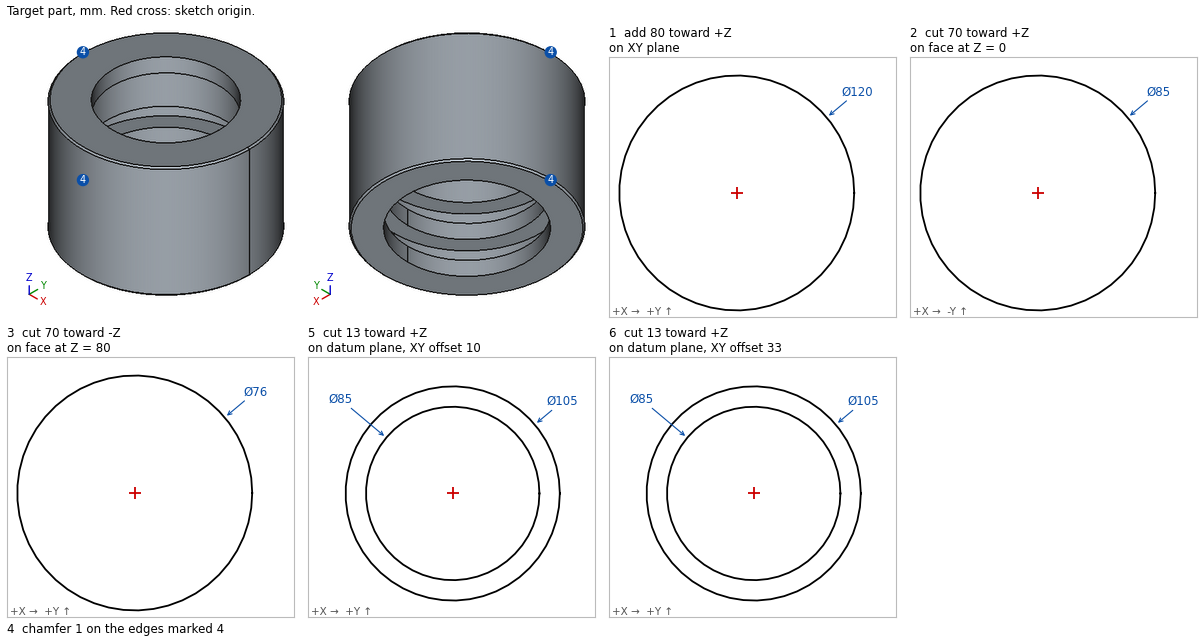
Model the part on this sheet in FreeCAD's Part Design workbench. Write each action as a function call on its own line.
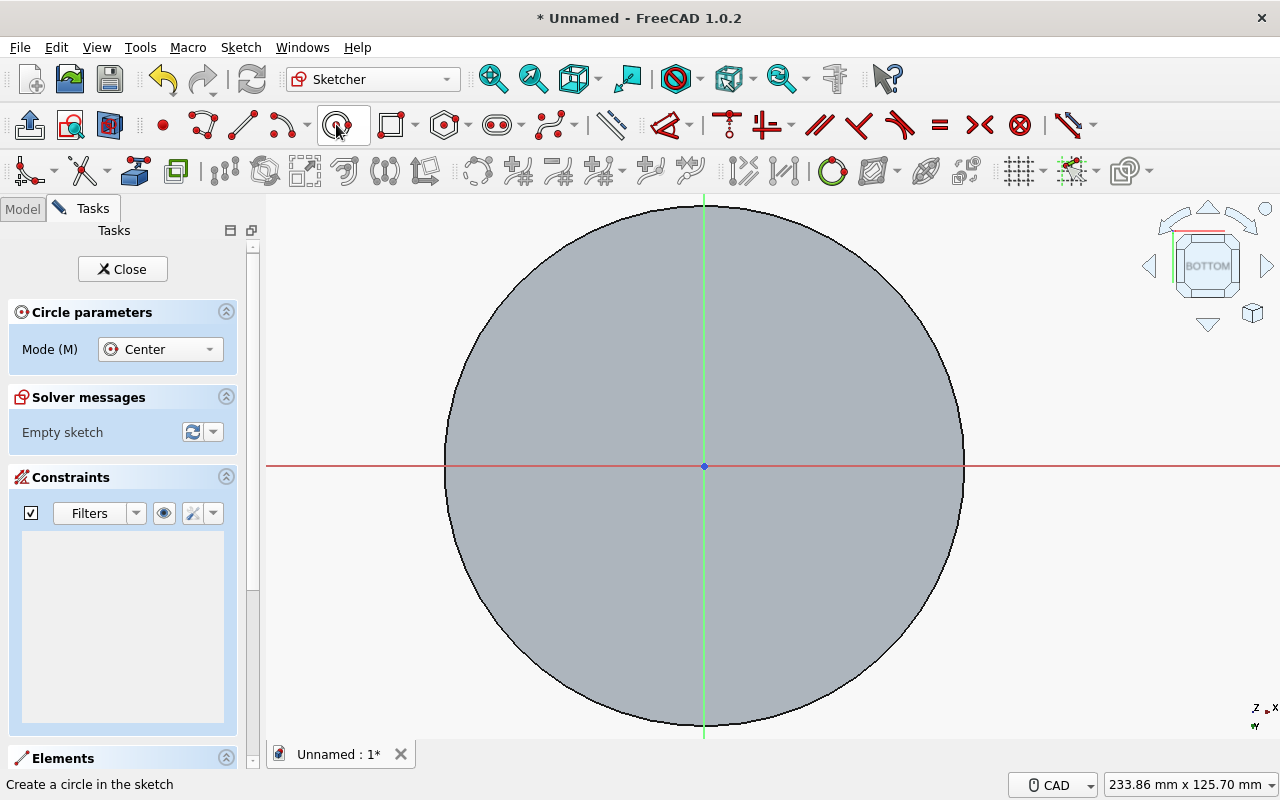
click(704, 466)
click(835, 336)
key(Escape)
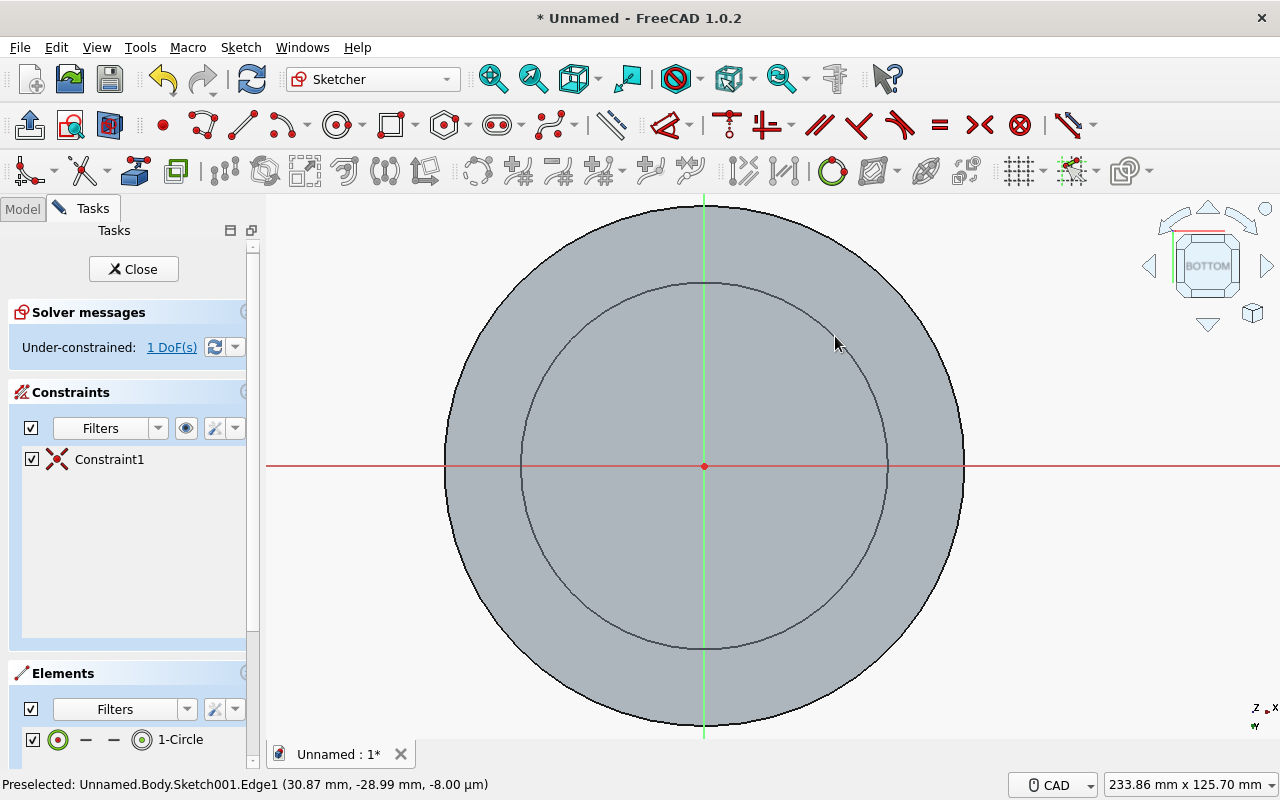
click(834, 336)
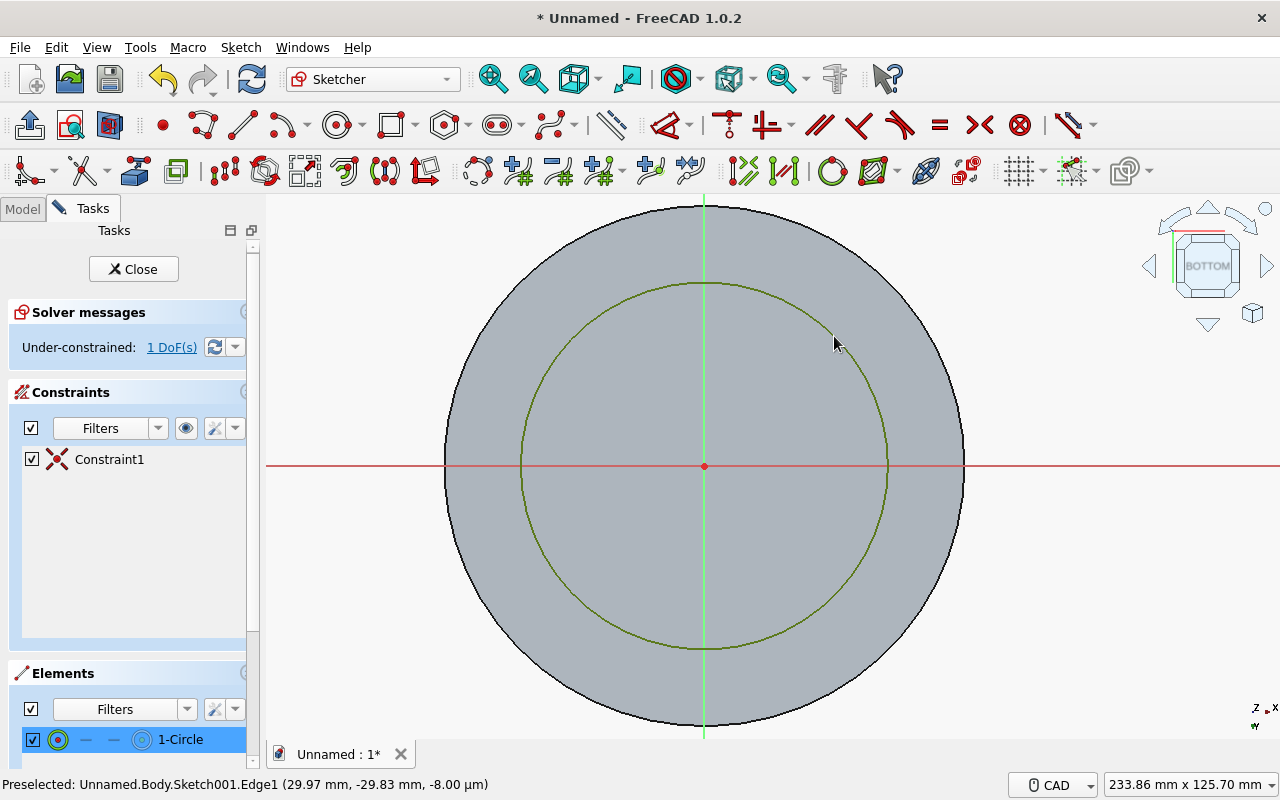
key(k)
key(o)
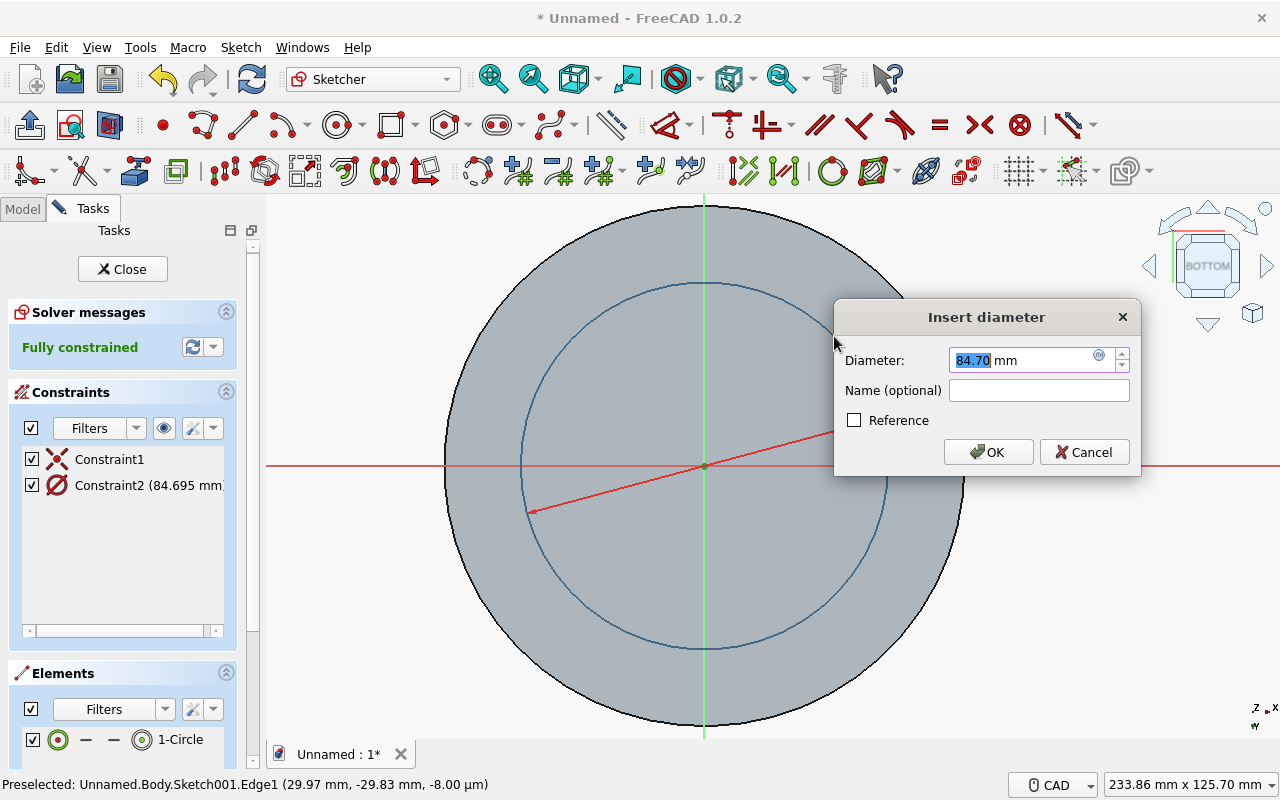
text(85)
key(Return)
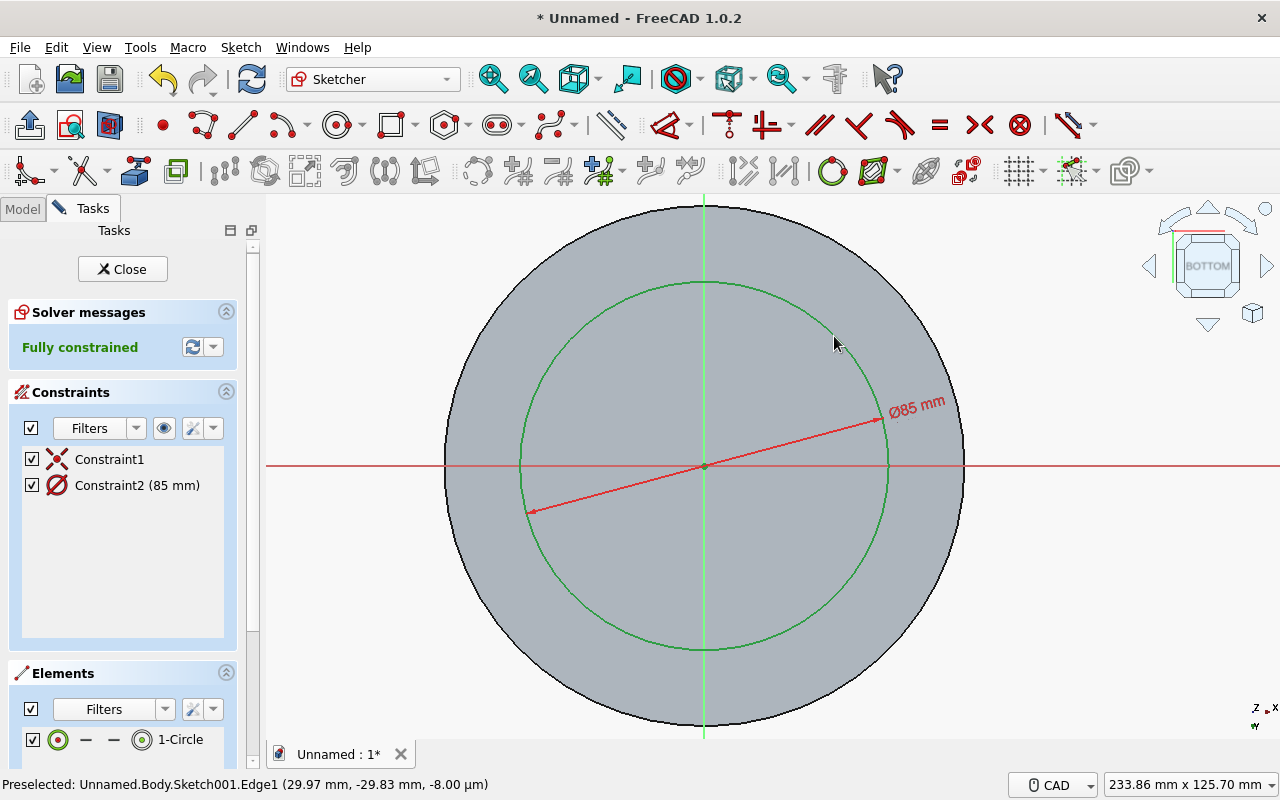
click(123, 269)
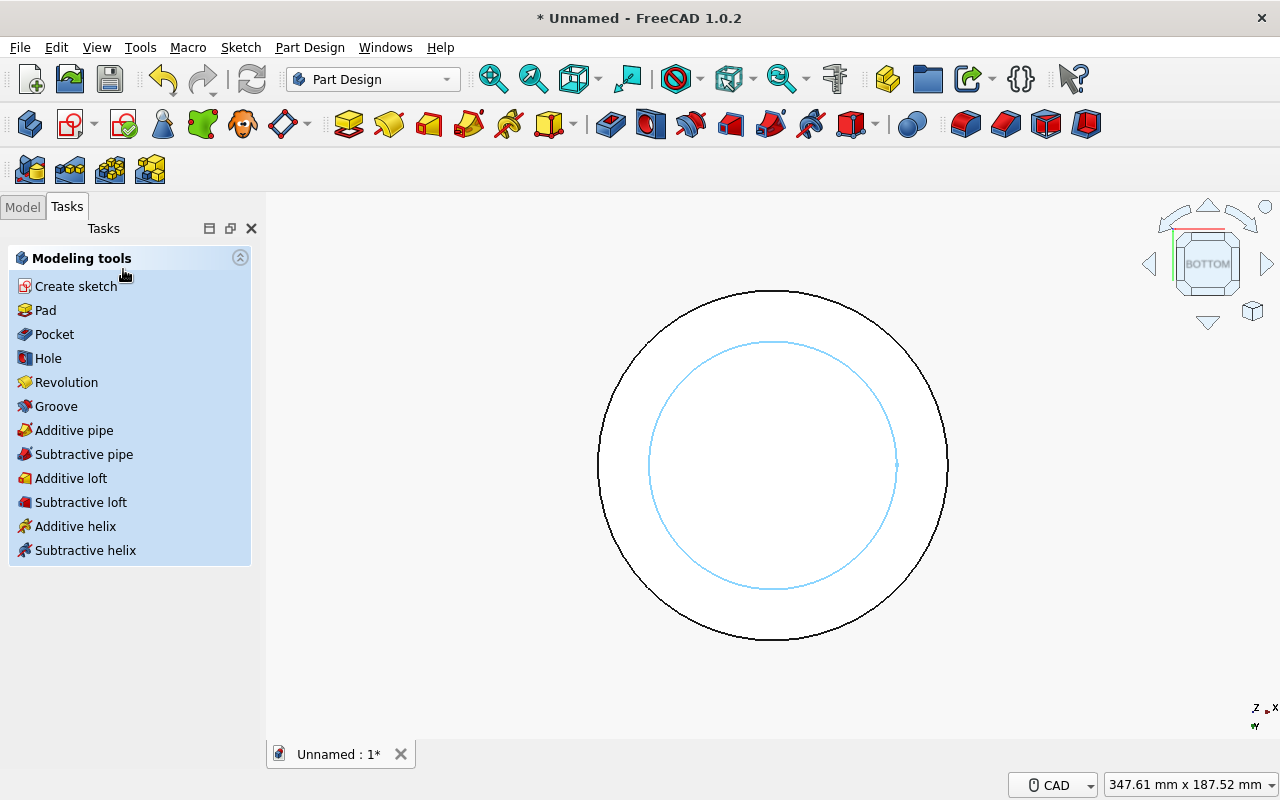
click(612, 124)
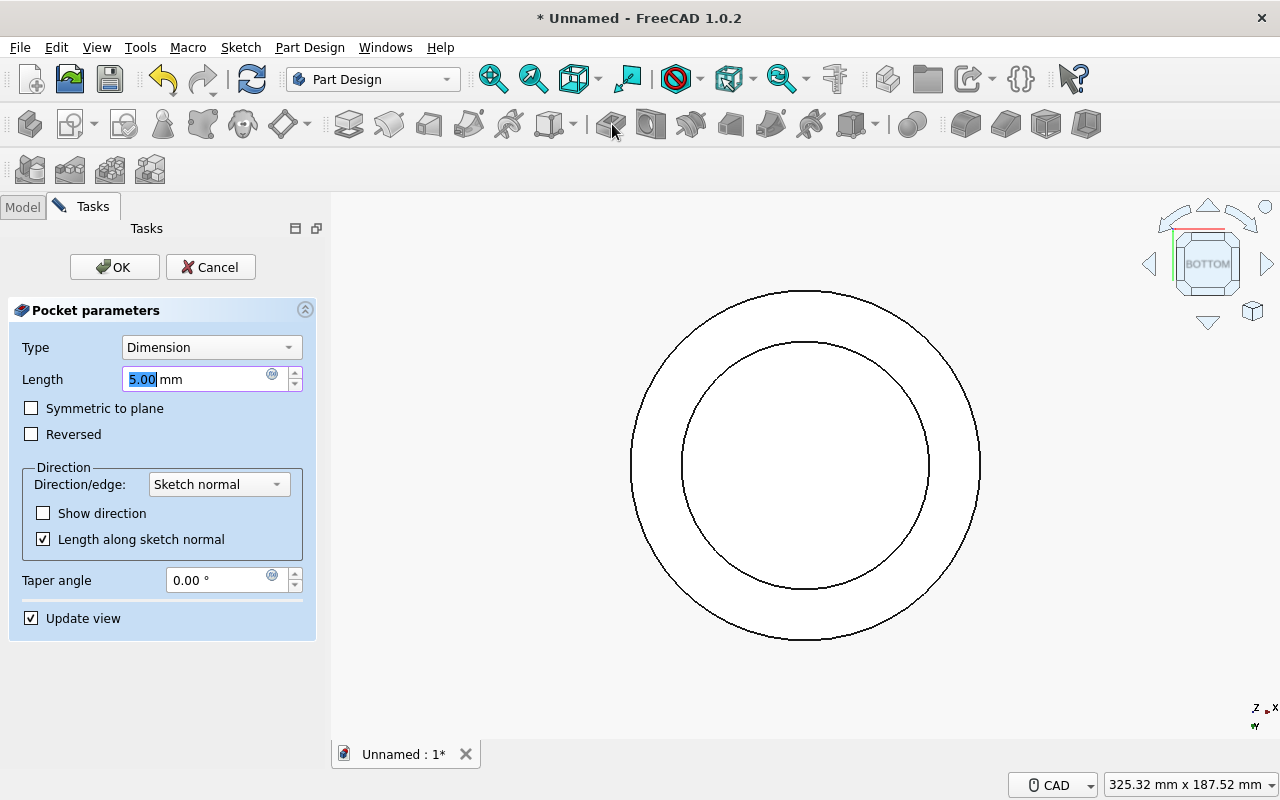
text(70)
key(Tab)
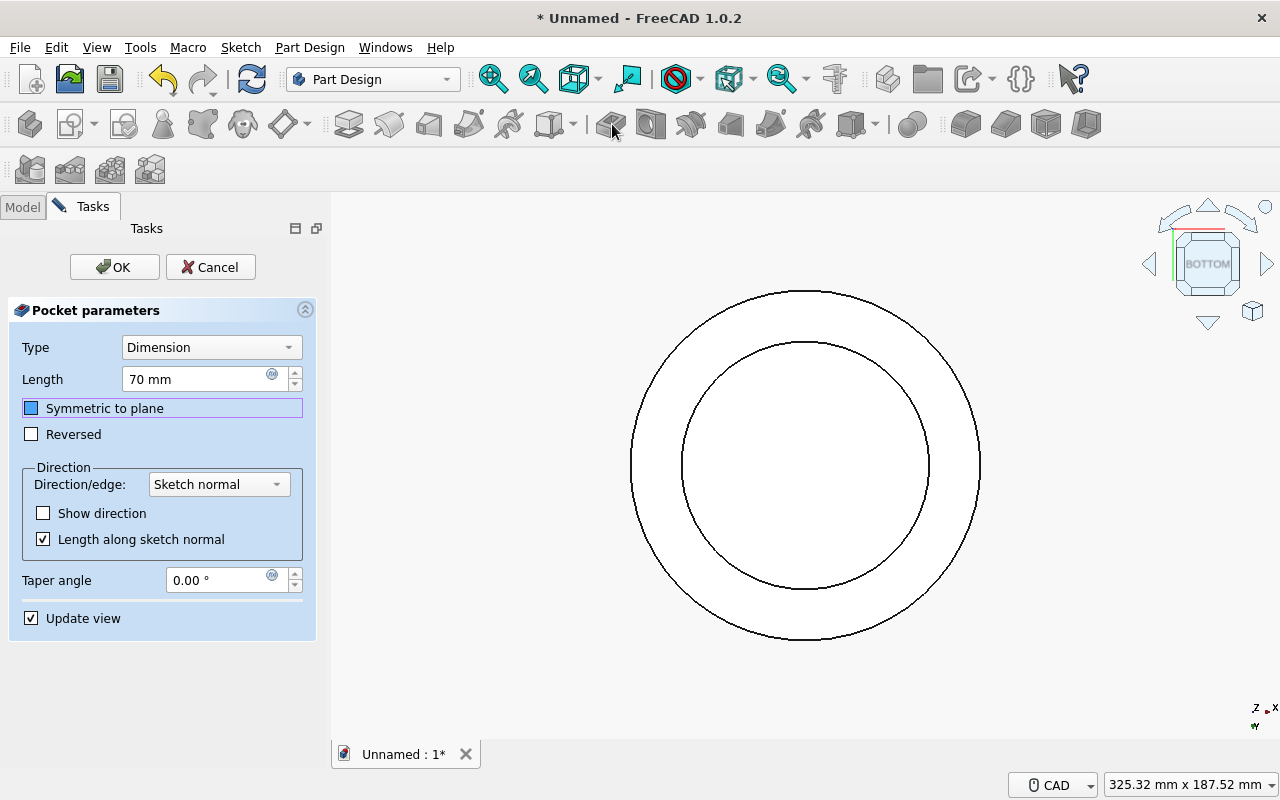
click(115, 267)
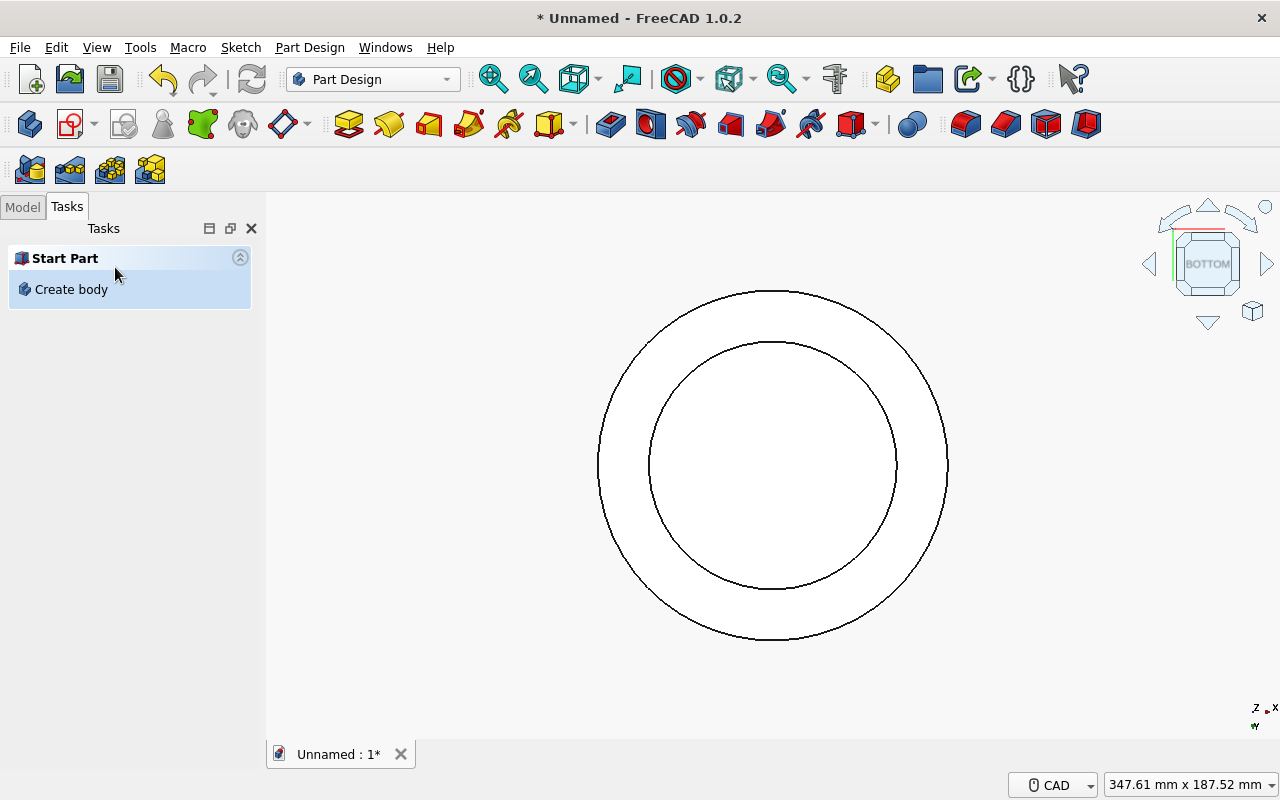
key(0)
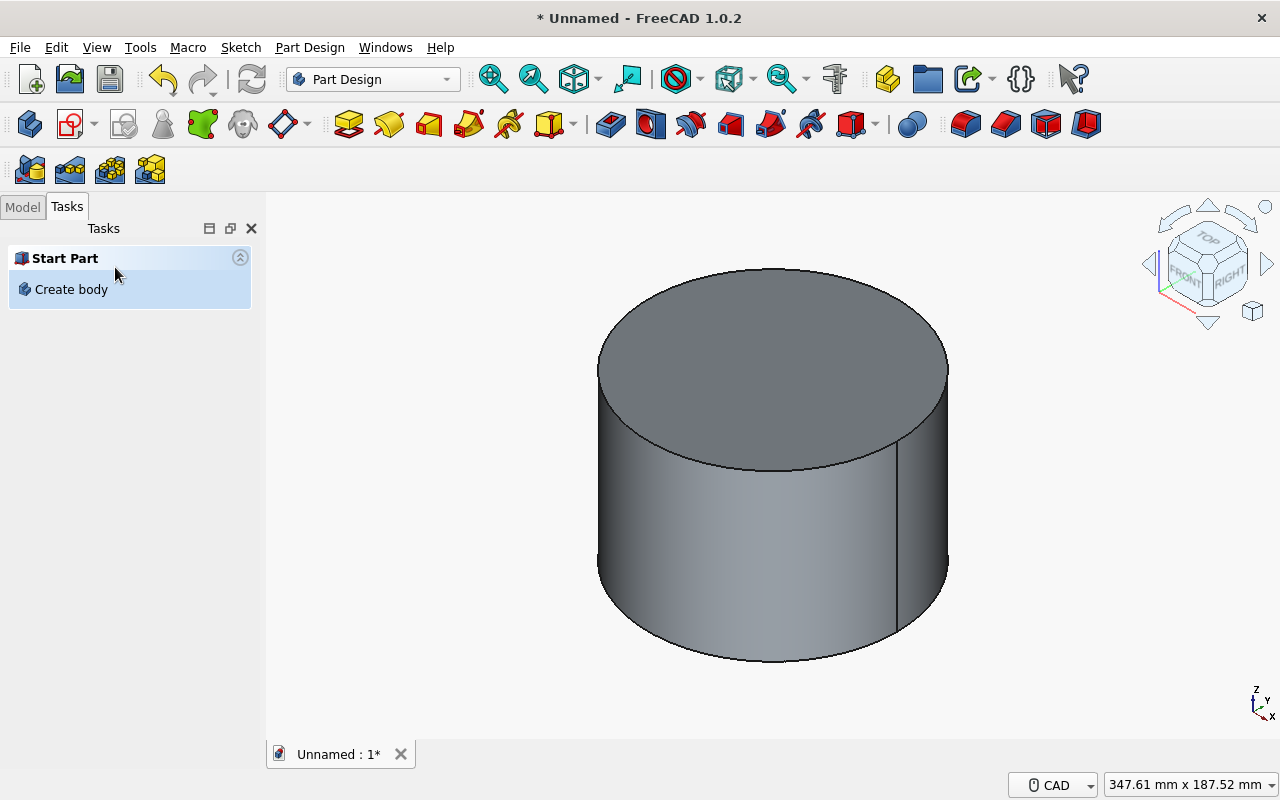
click(773, 369)